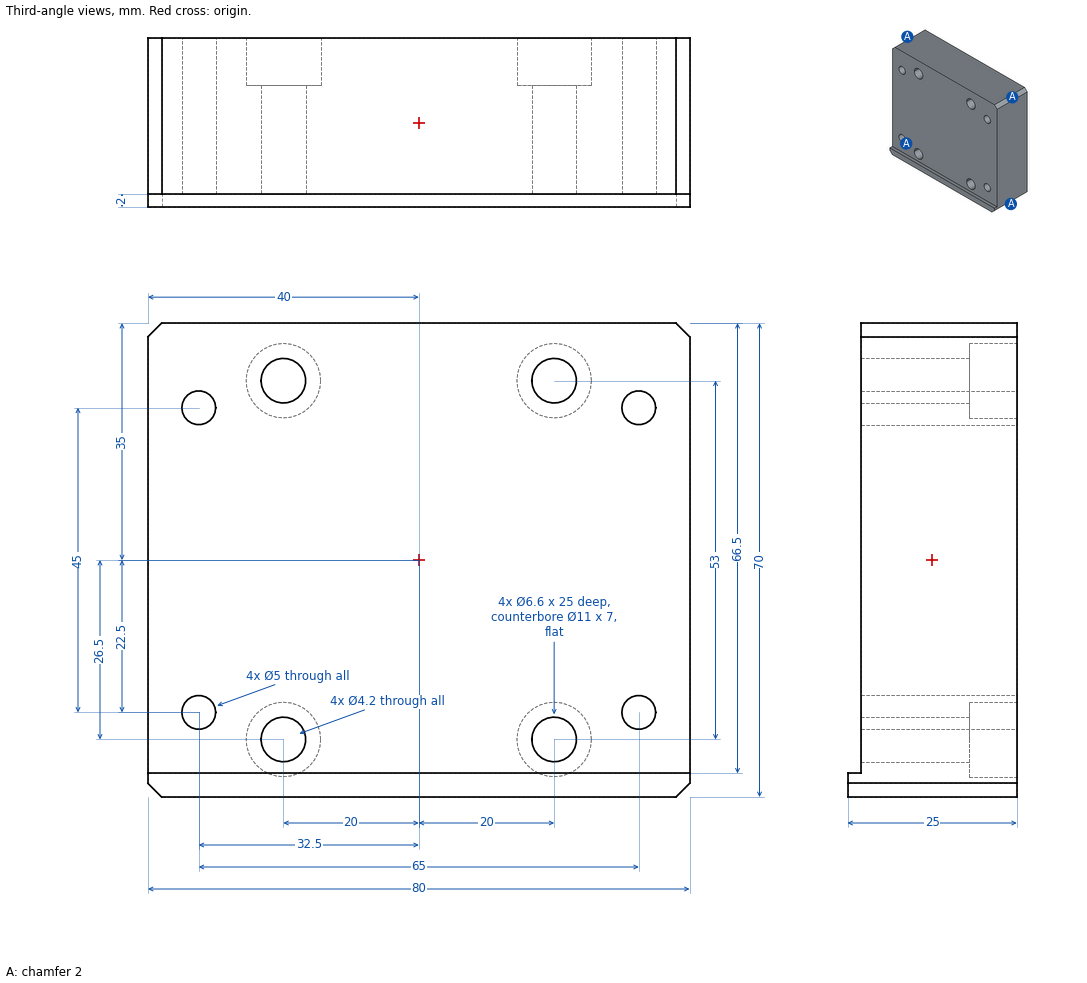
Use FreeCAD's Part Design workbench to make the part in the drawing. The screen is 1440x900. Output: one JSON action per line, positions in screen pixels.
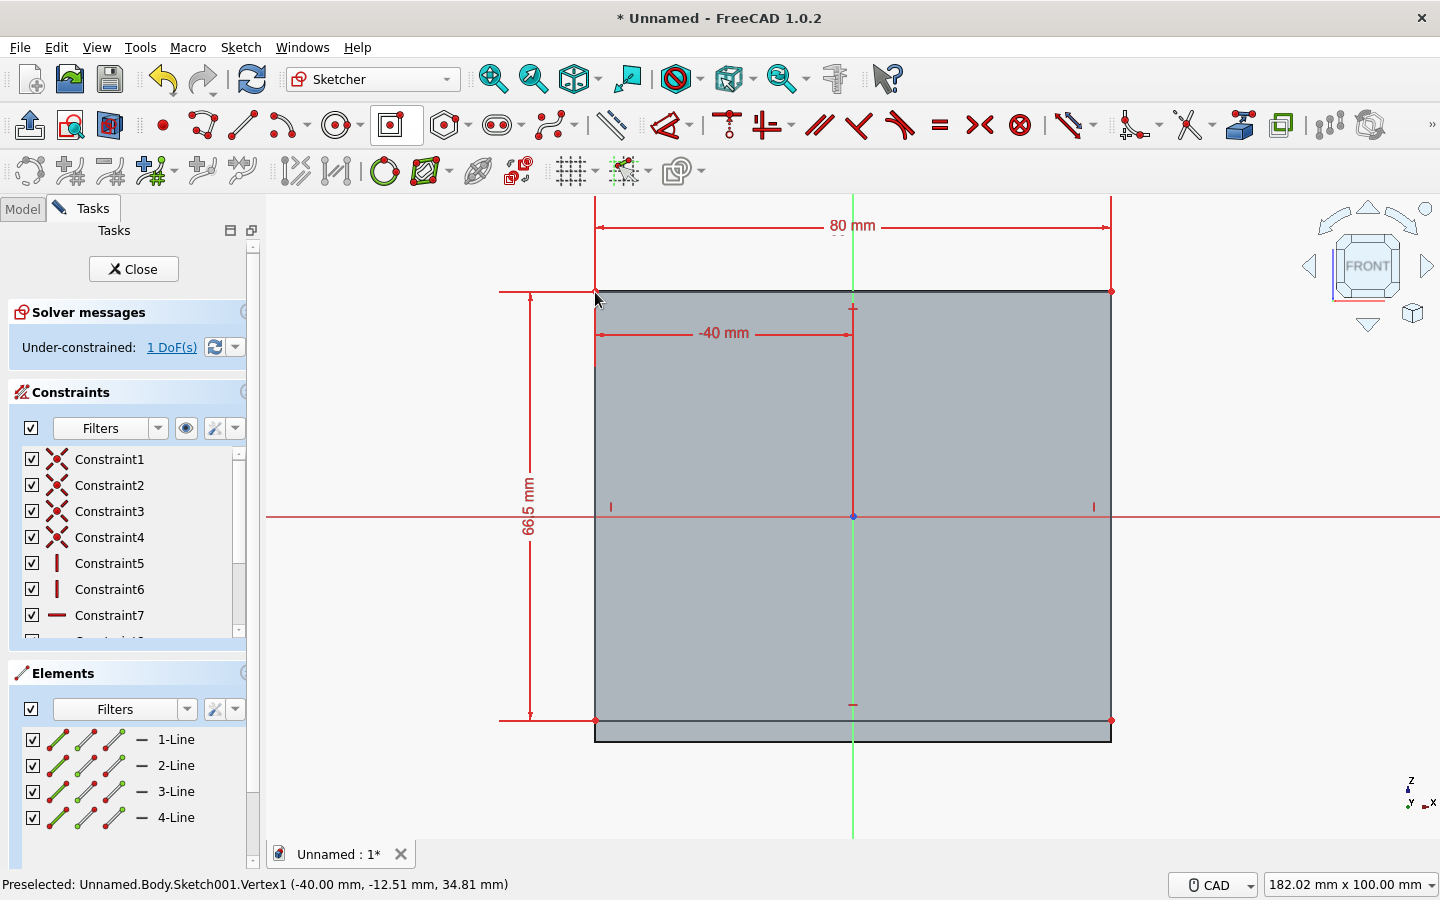
{"action": "left_click", "coordinate": [595, 292]}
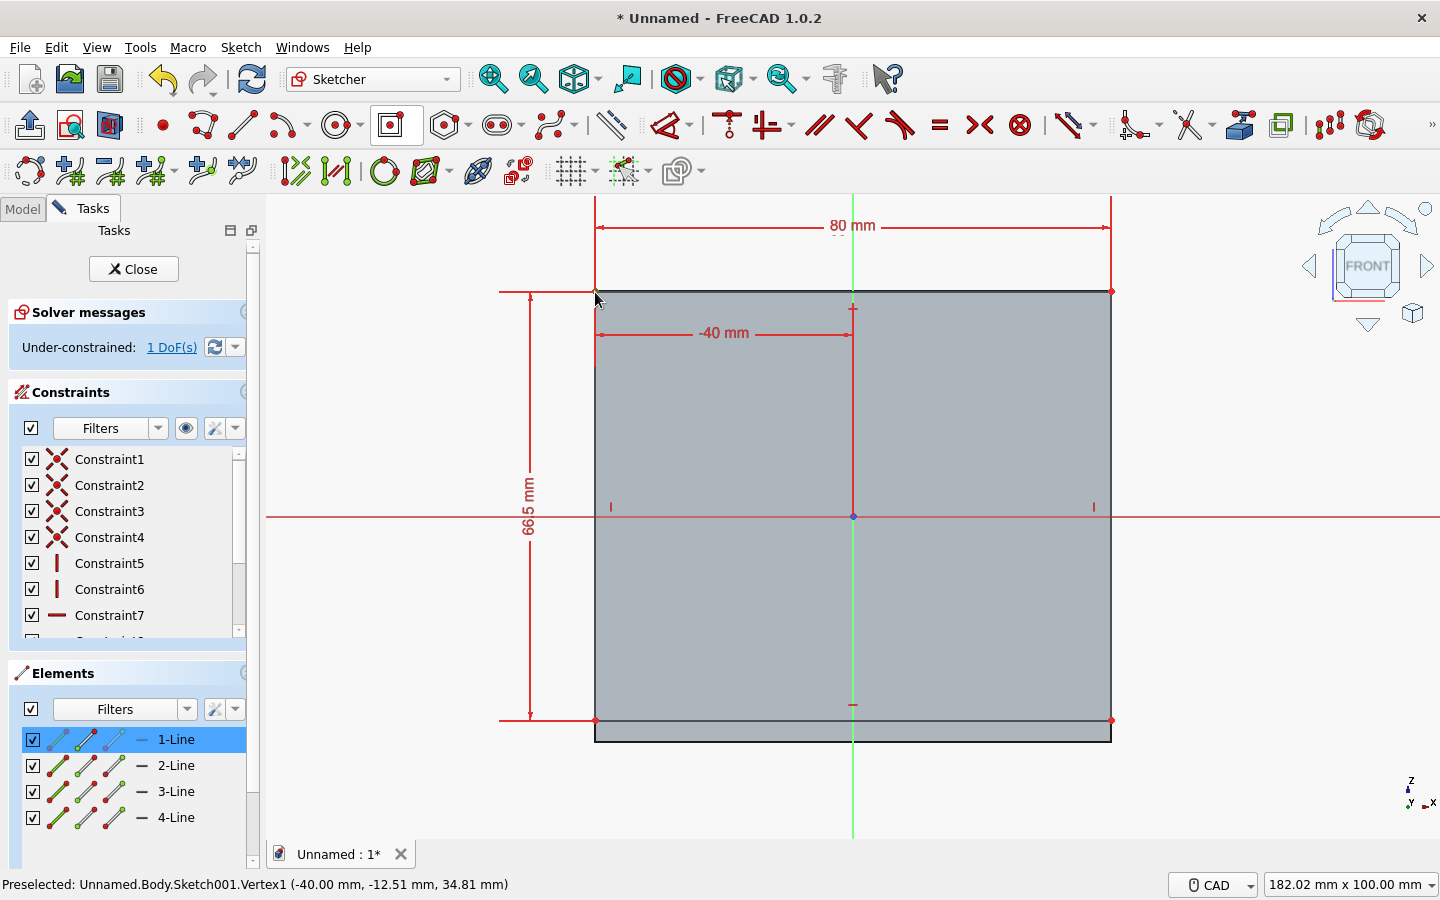
{"action": "left_click", "coordinate": [692, 126]}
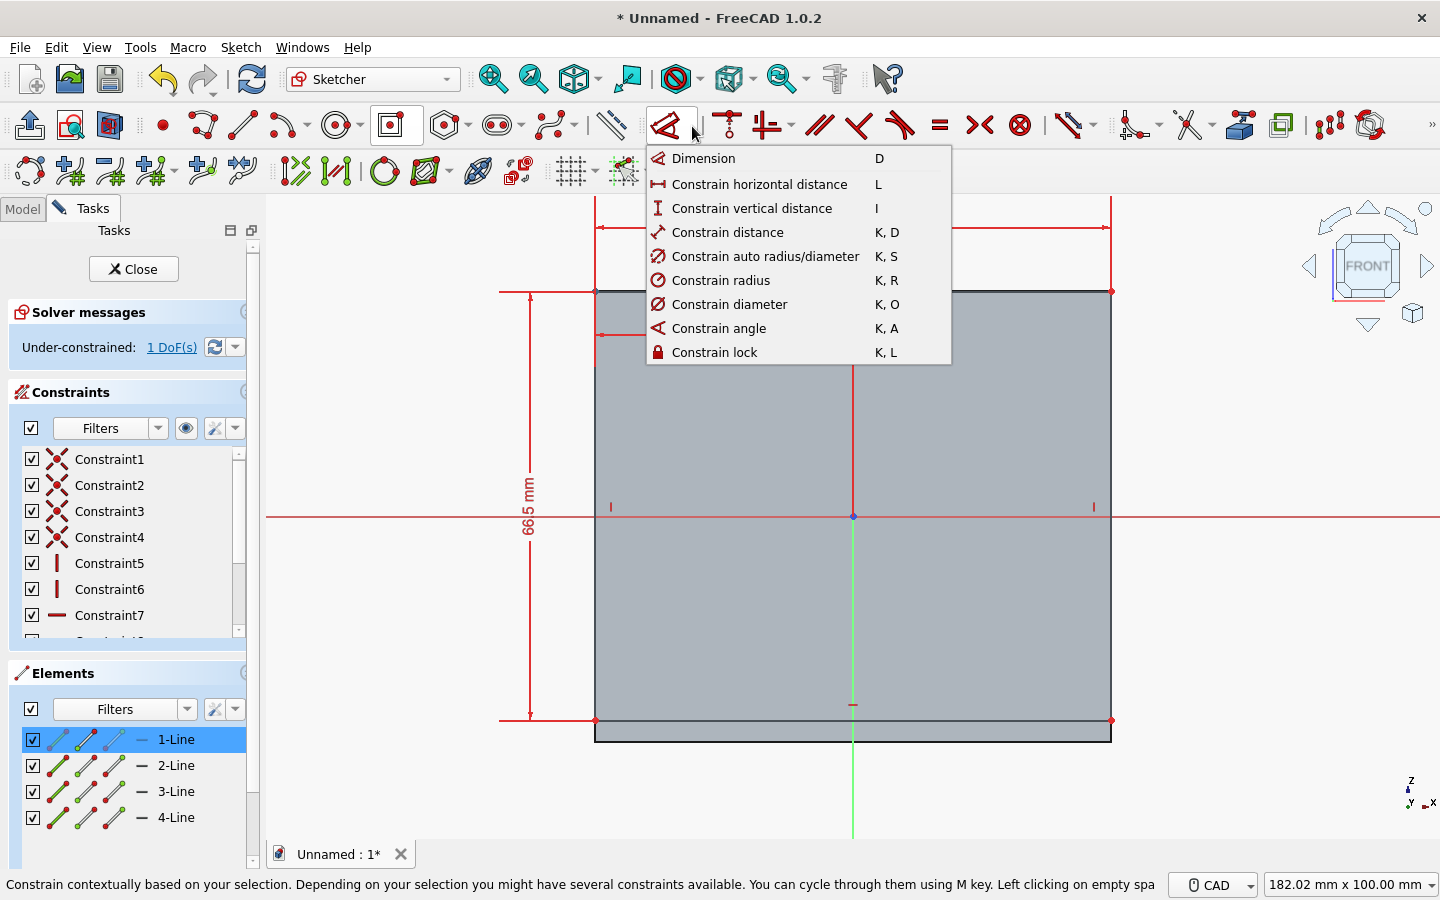
{"action": "left_click", "coordinate": [799, 208]}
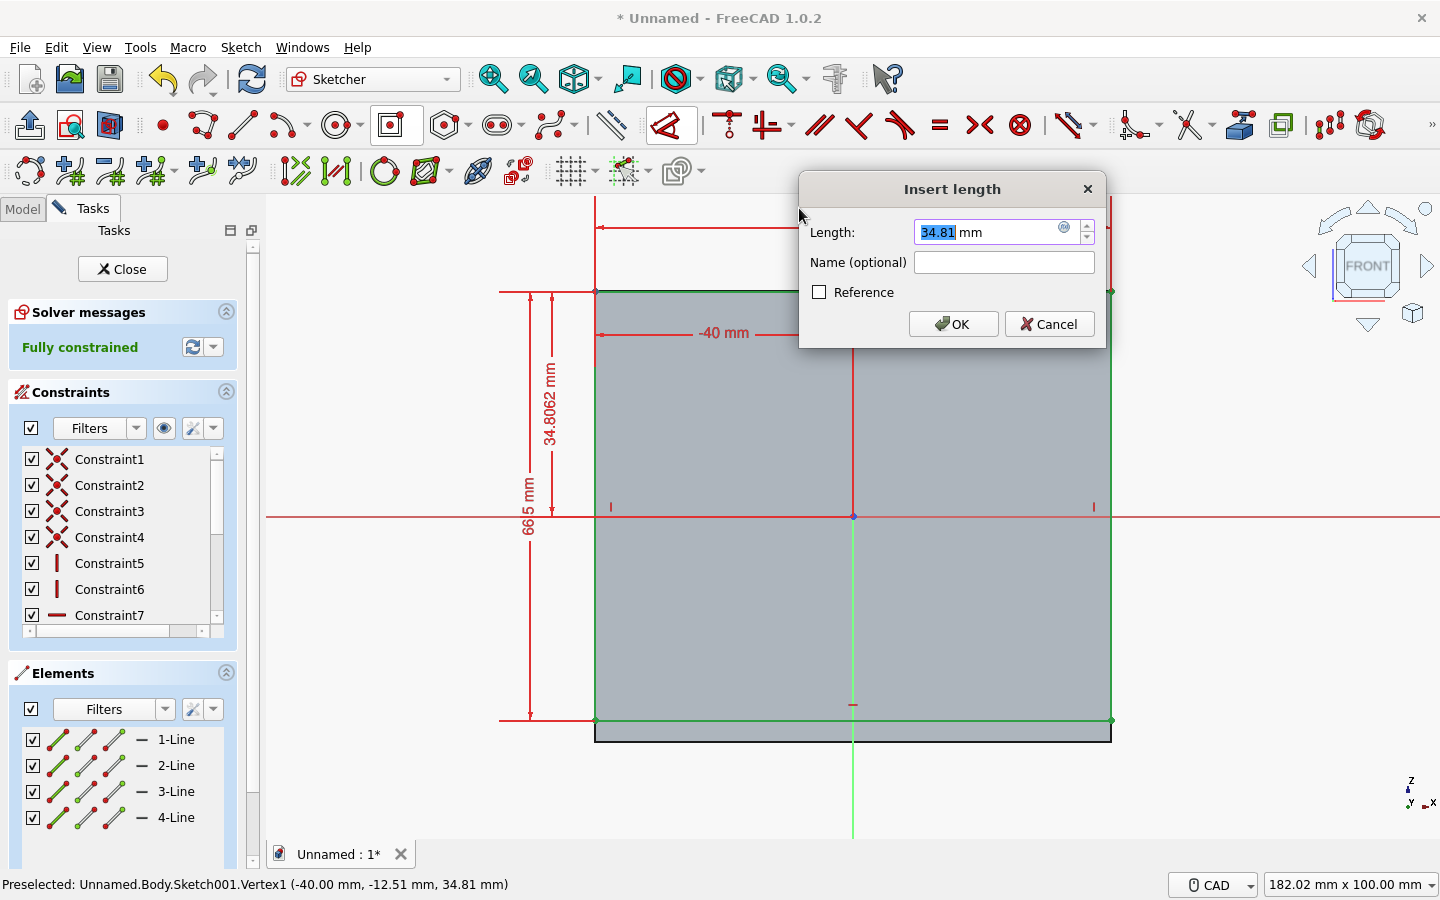
{"action": "type", "text": "35"}
{"action": "key", "text": "Return"}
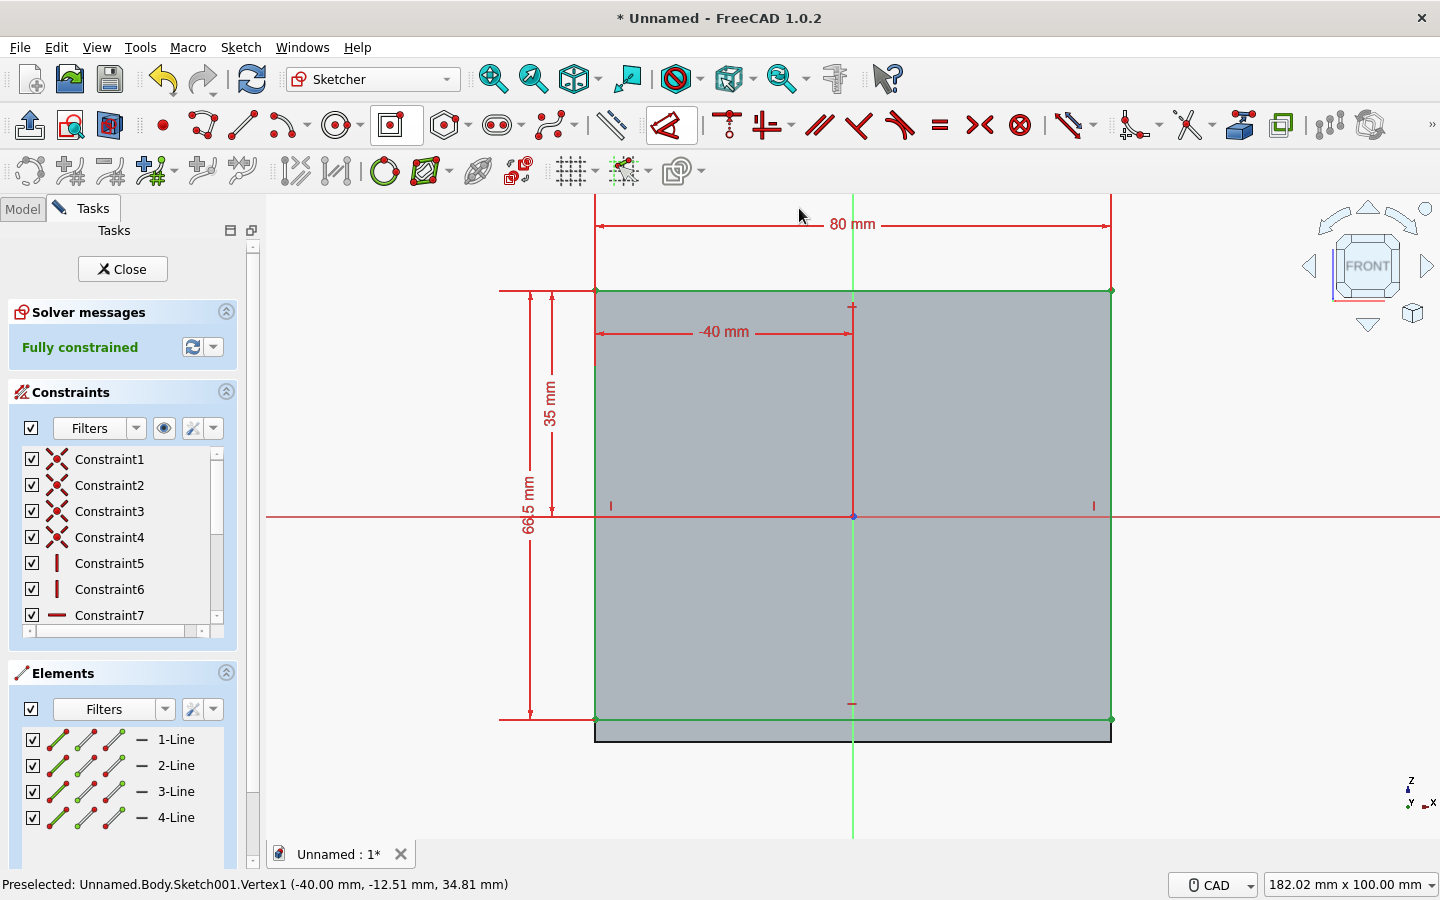
{"action": "left_click", "coordinate": [123, 269]}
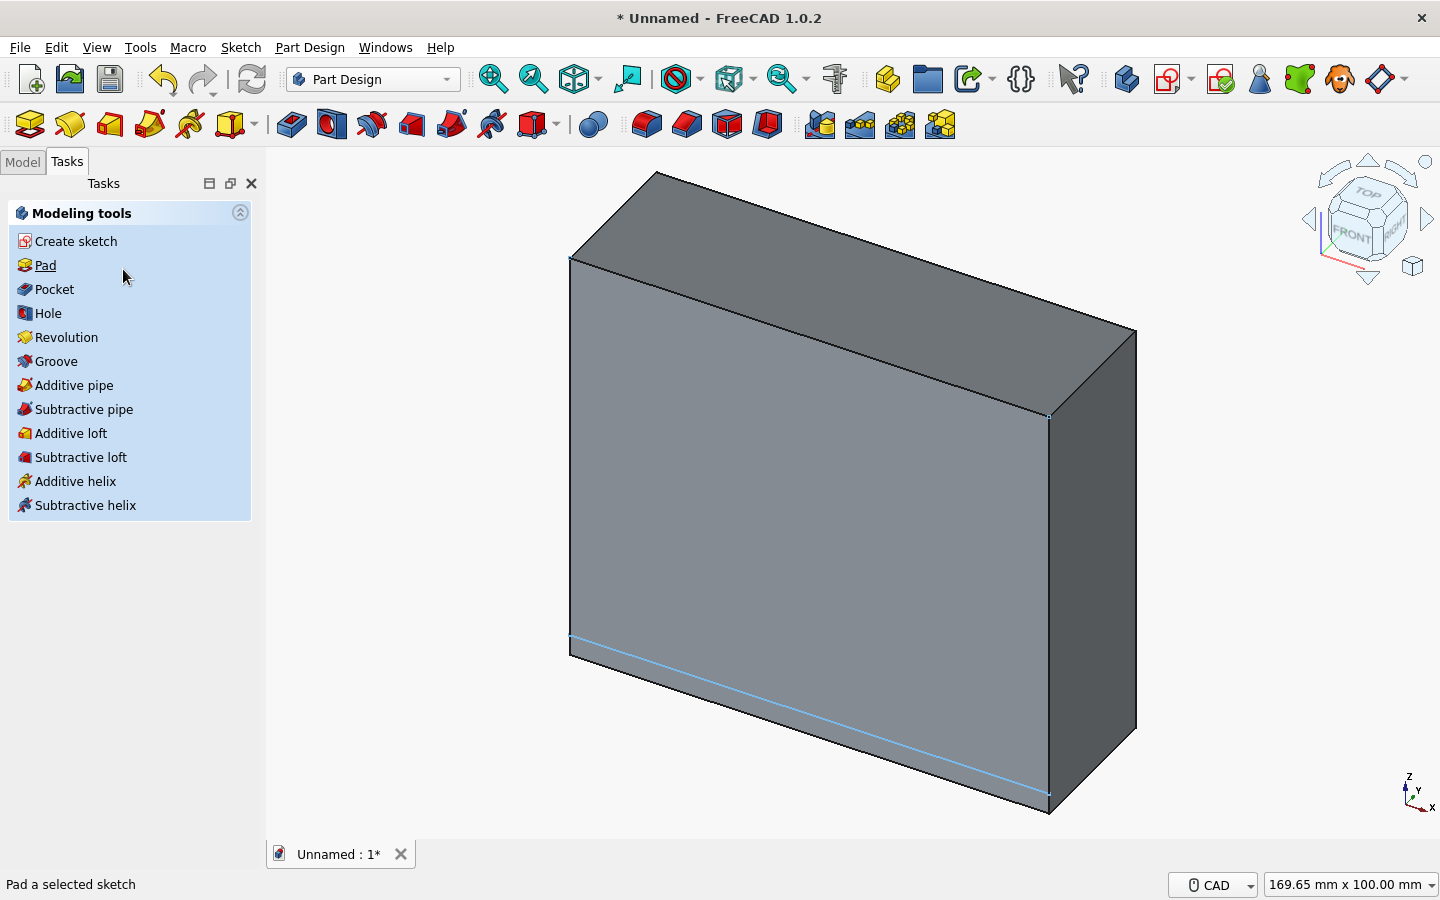
{"action": "left_click", "coordinate": [292, 124]}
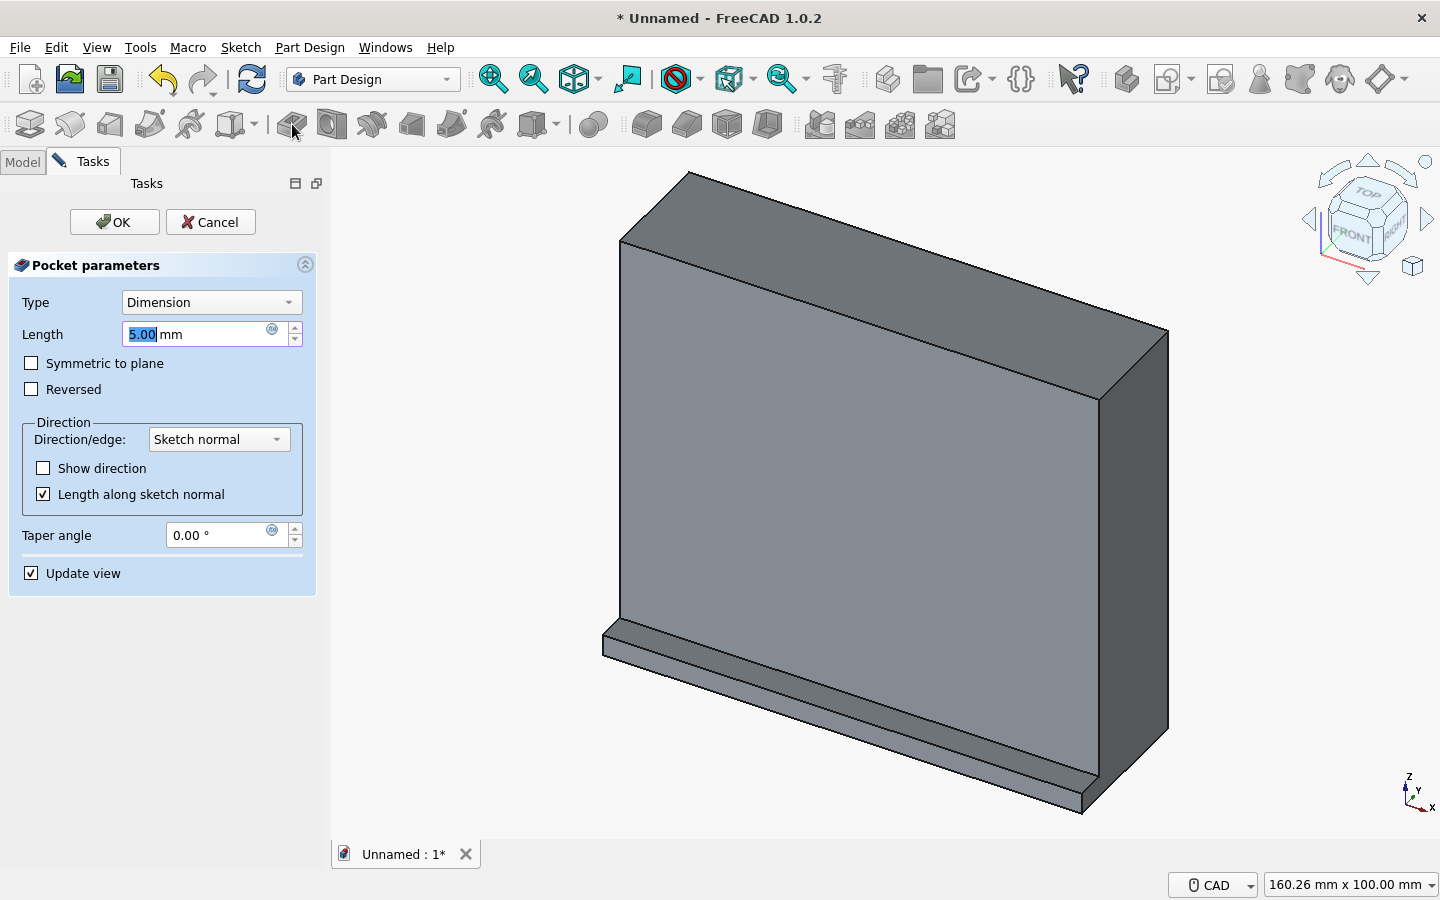
{"action": "type", "text": "2"}
{"action": "key", "text": "Tab"}